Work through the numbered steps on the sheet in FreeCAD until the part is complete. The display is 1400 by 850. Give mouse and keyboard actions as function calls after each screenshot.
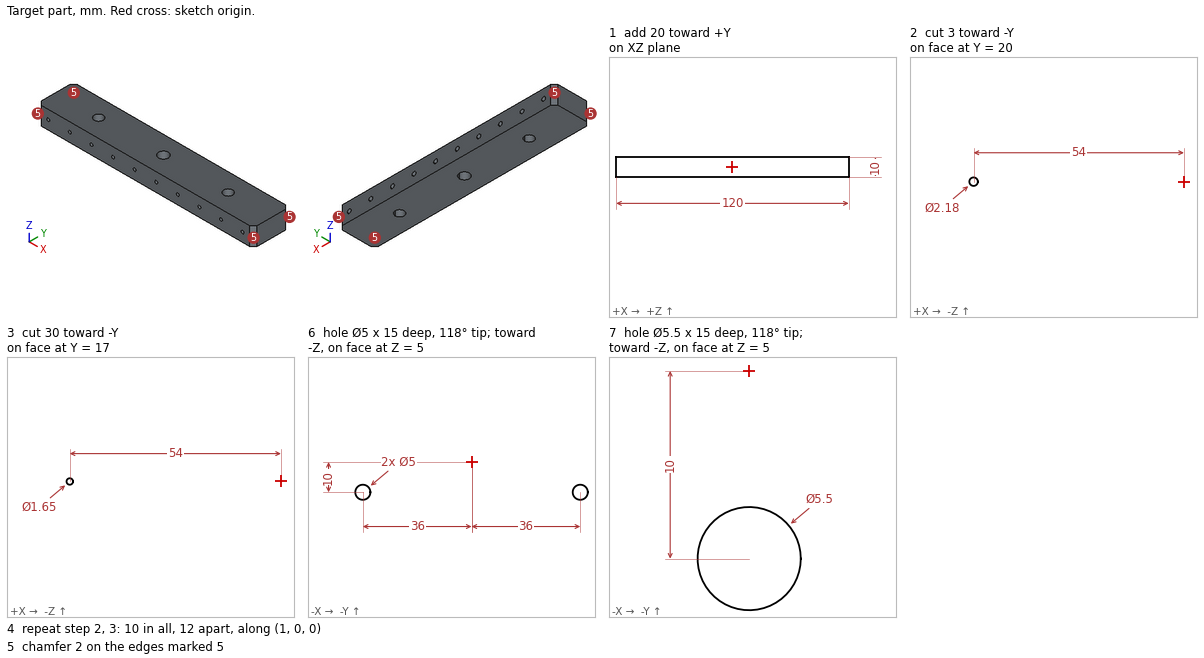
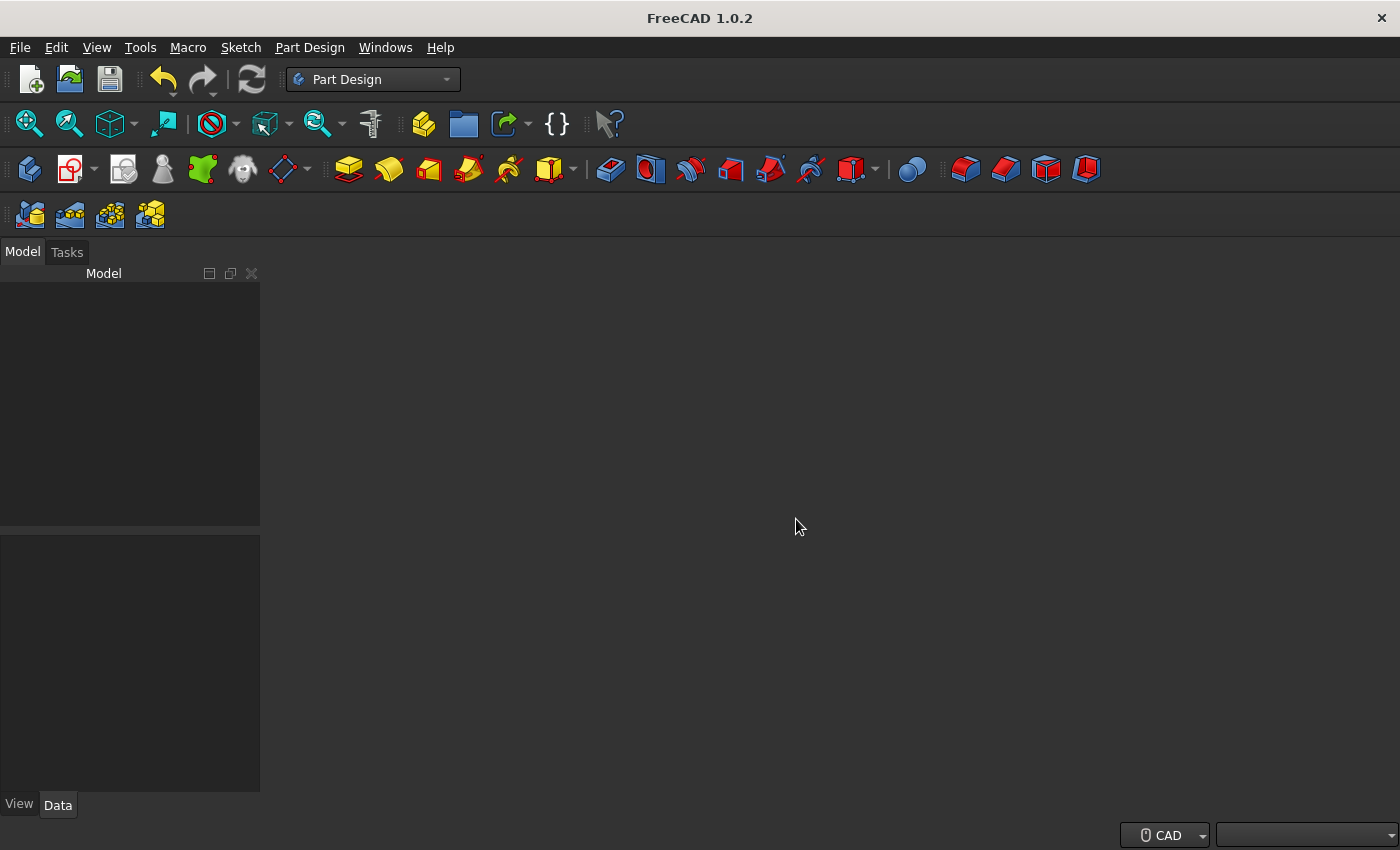
click(30, 80)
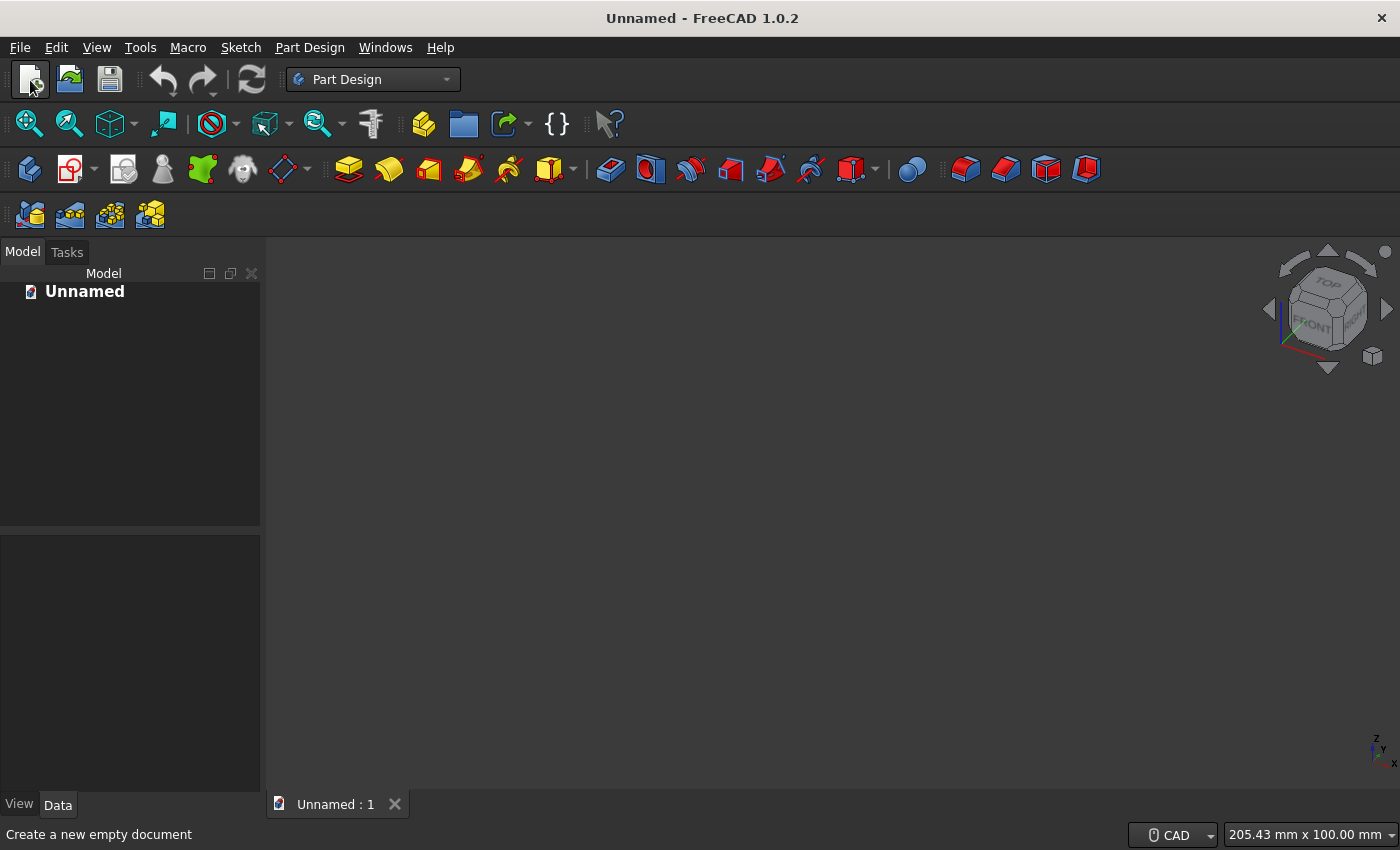
click(70, 170)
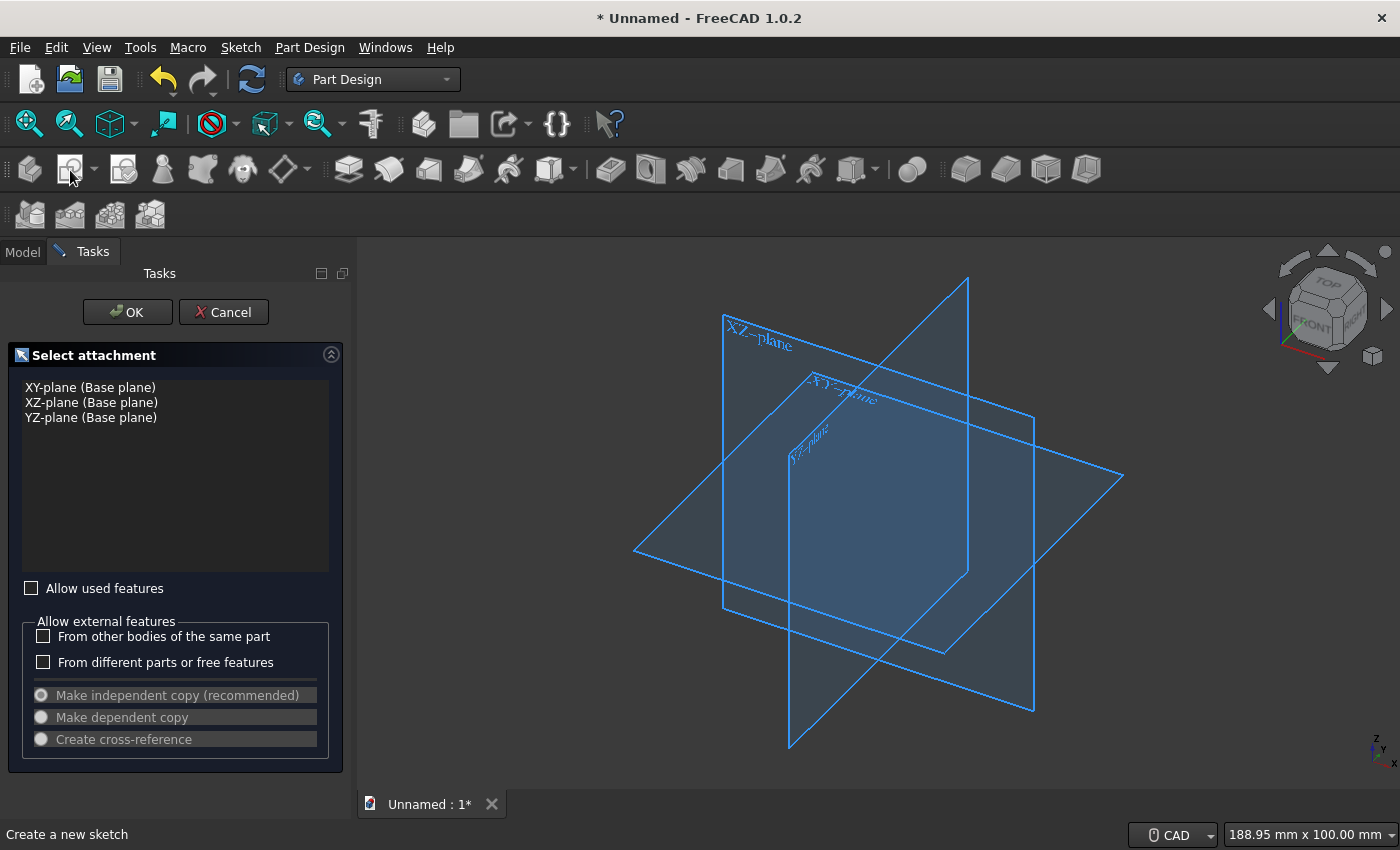
click(82, 402)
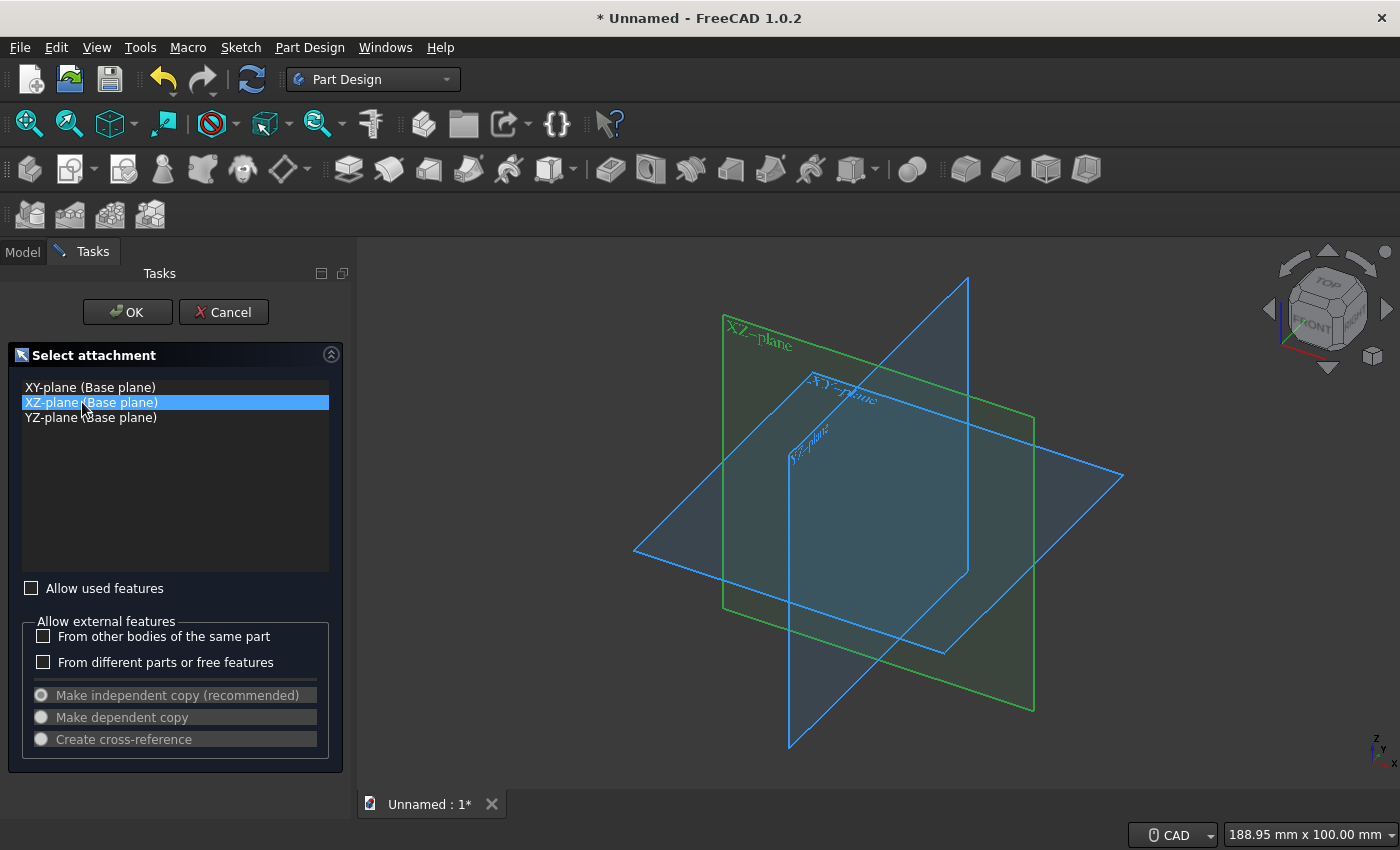
click(128, 312)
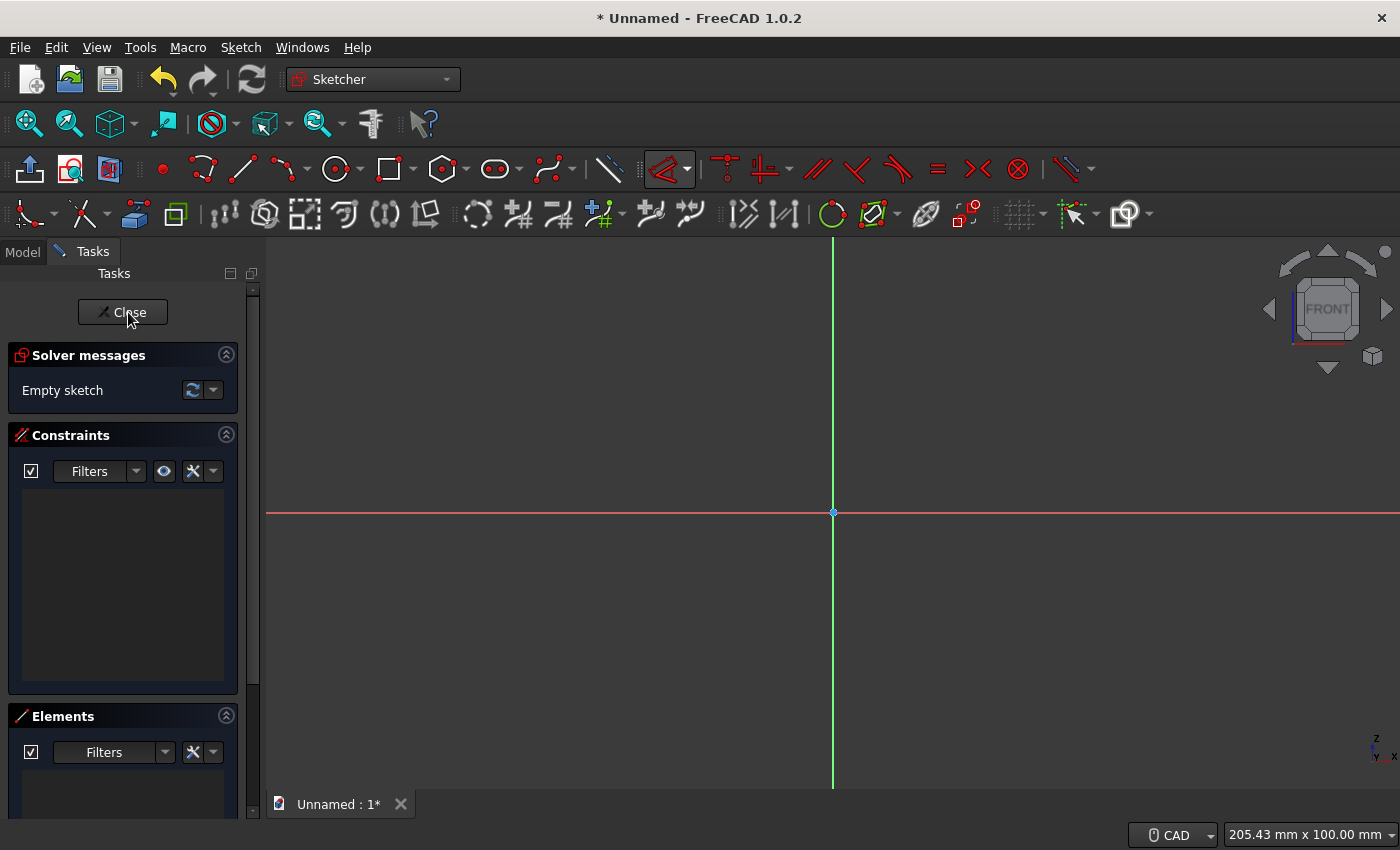
key(g)
key(v)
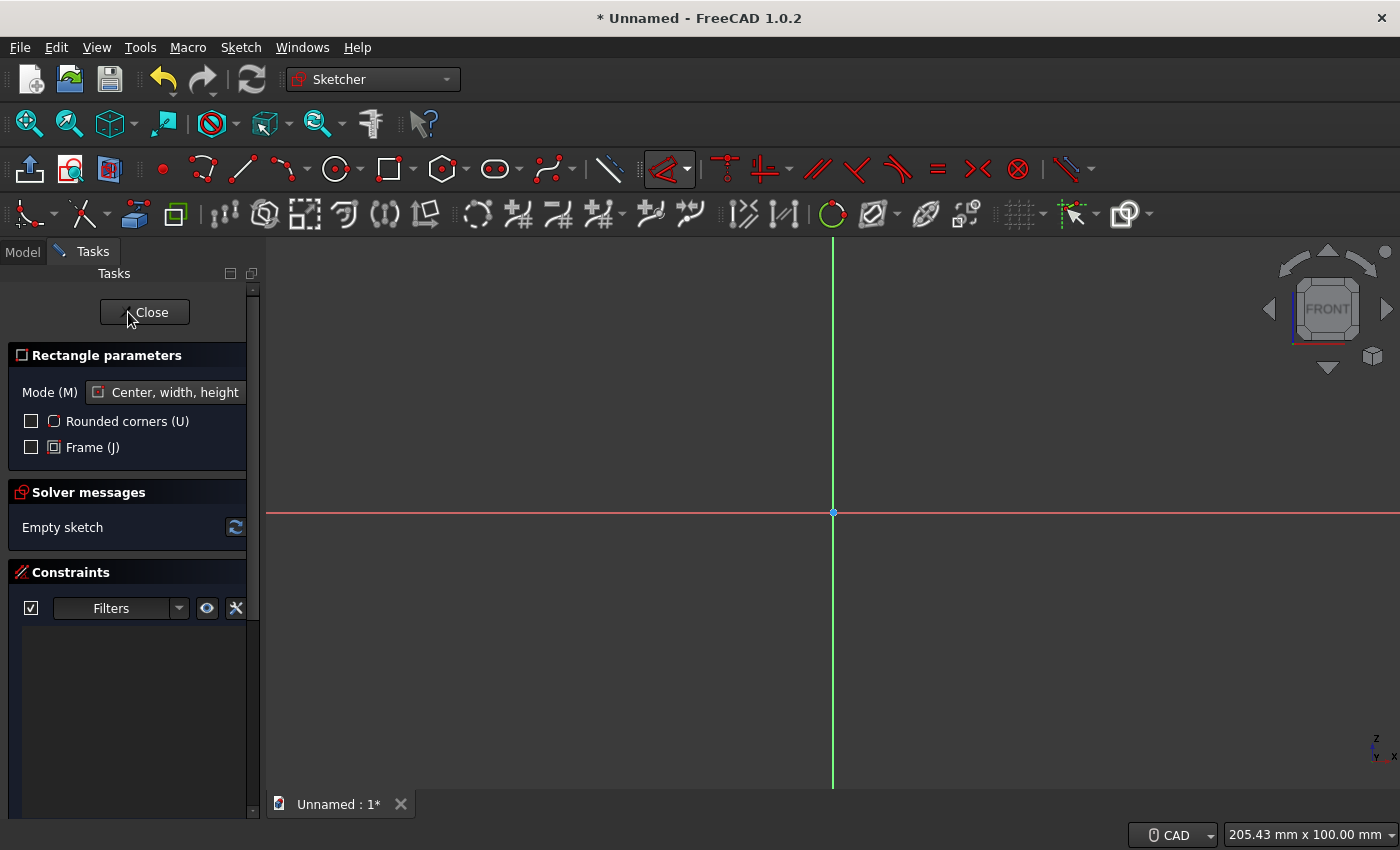
click(833, 513)
click(1164, 485)
key(Escape)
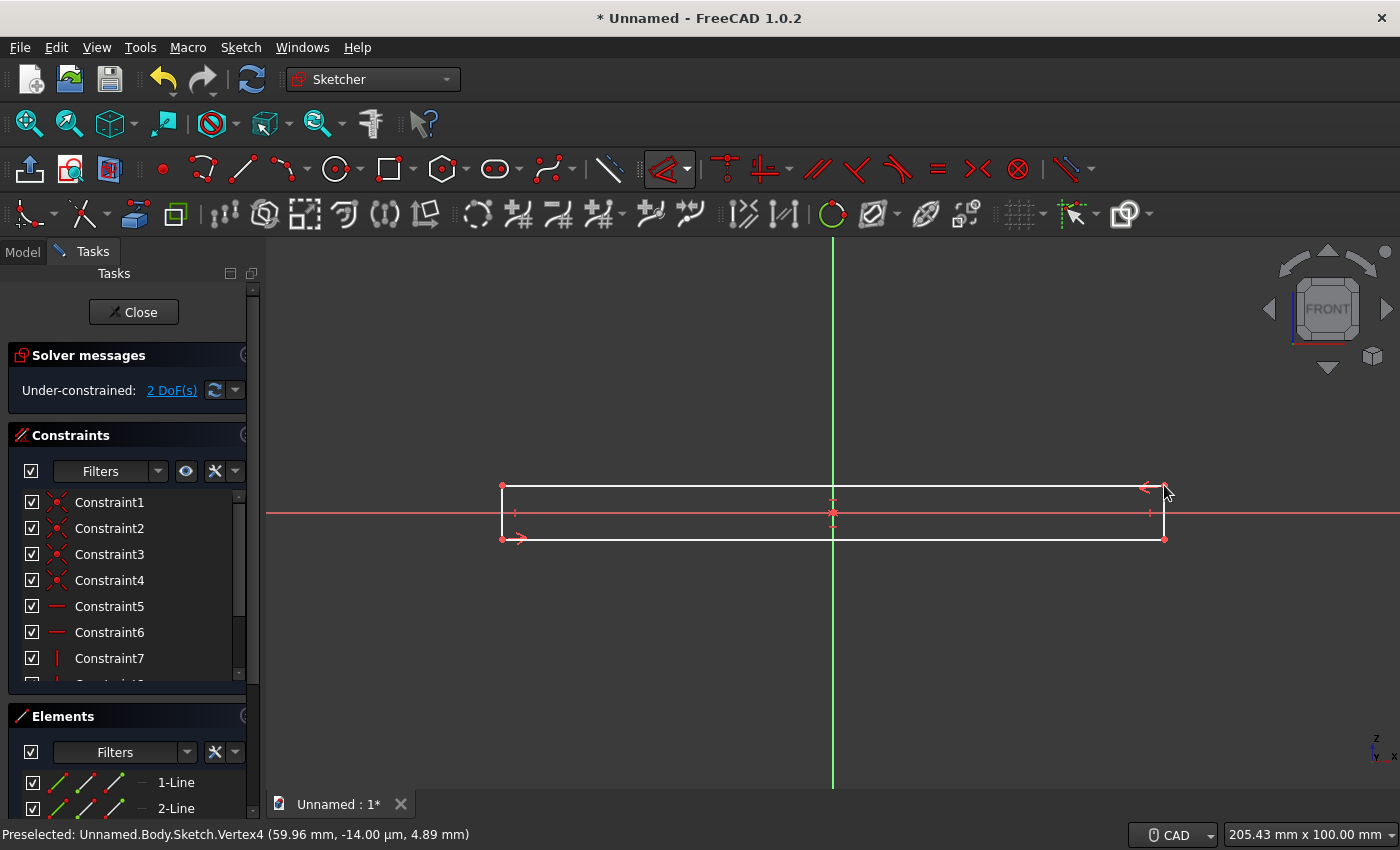
scroll(1164, 524, up, 2)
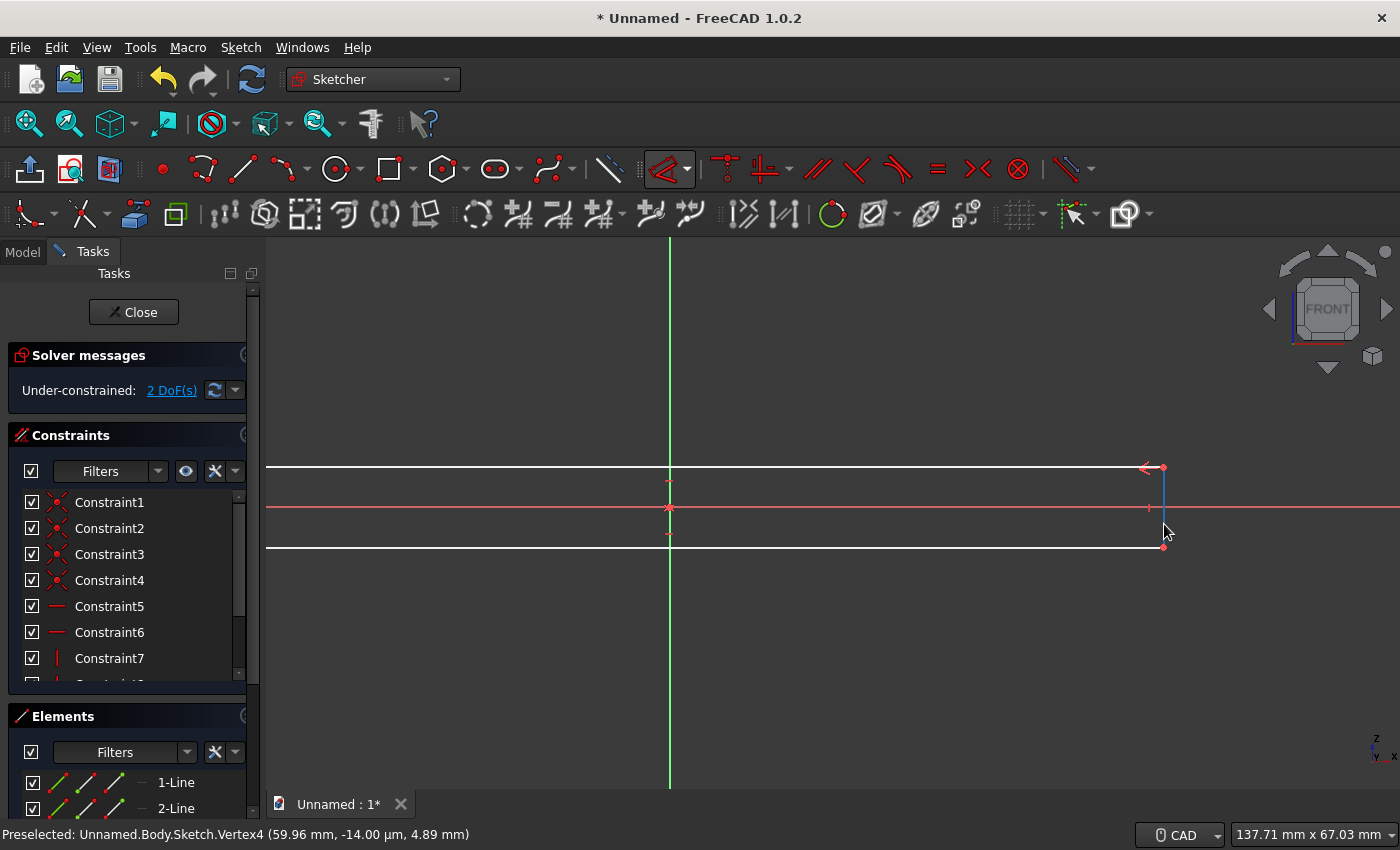
click(1164, 523)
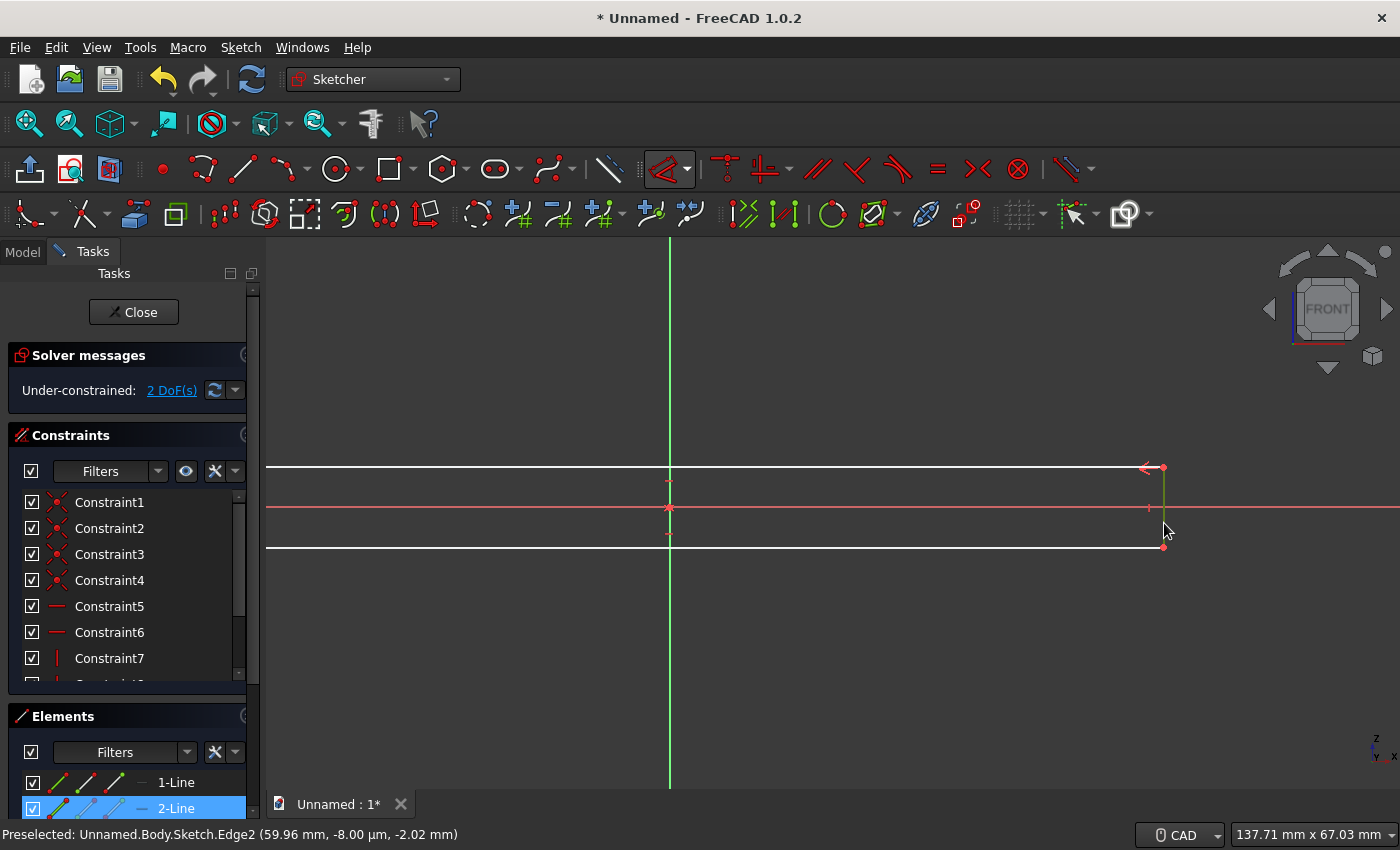
key(i)